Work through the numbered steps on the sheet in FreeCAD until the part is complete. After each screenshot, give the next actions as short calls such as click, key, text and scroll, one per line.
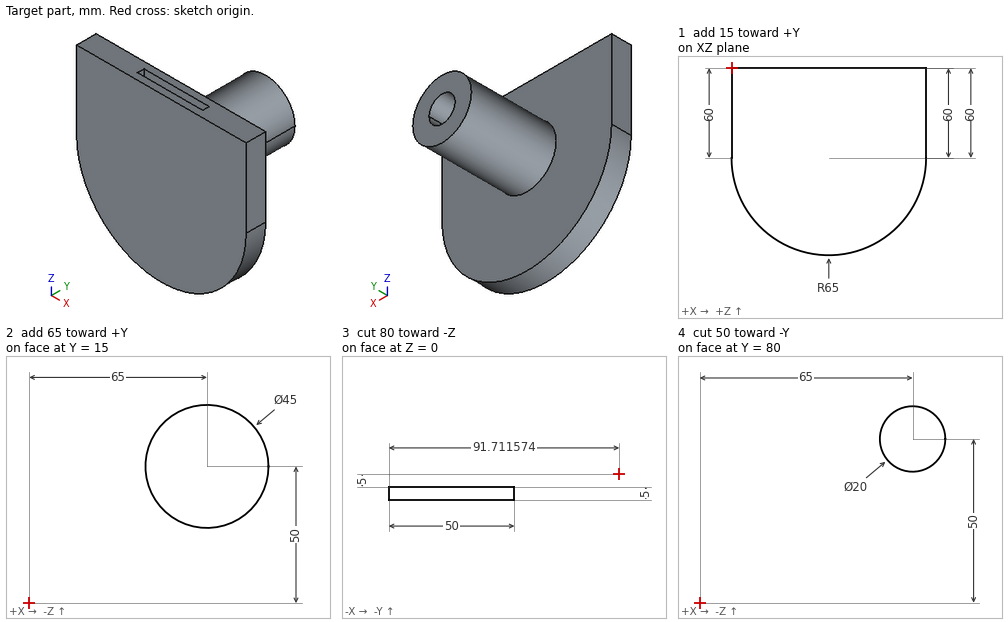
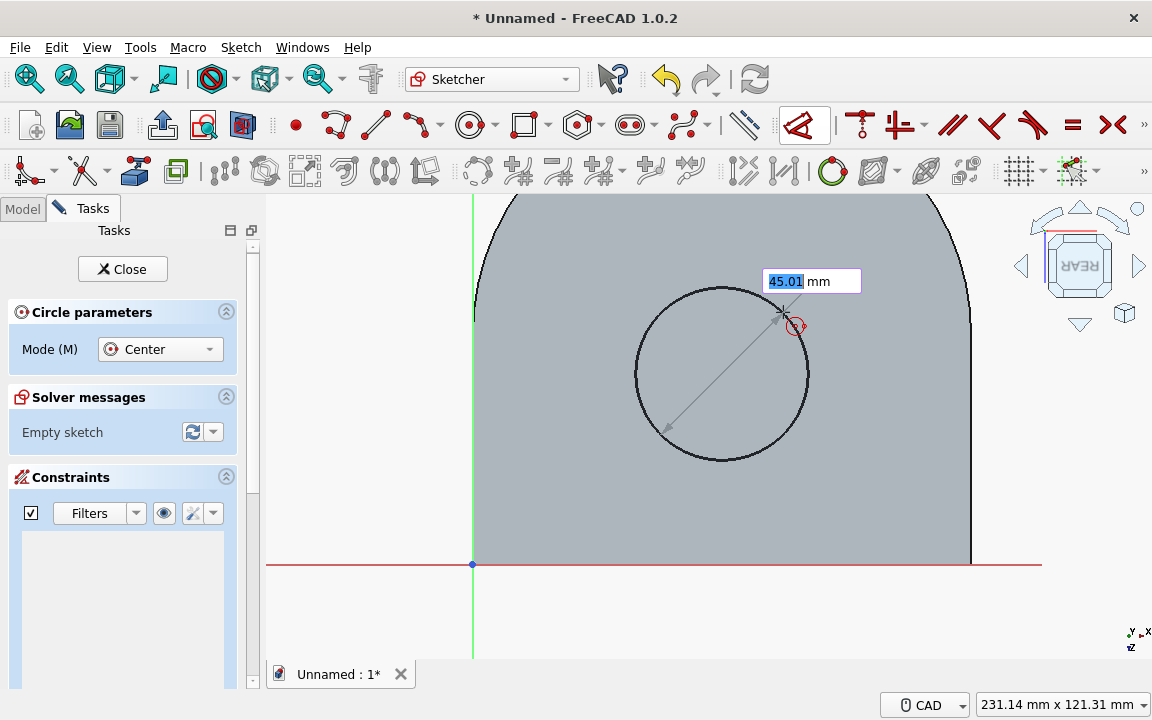
text(45)
key(Return)
key(Escape)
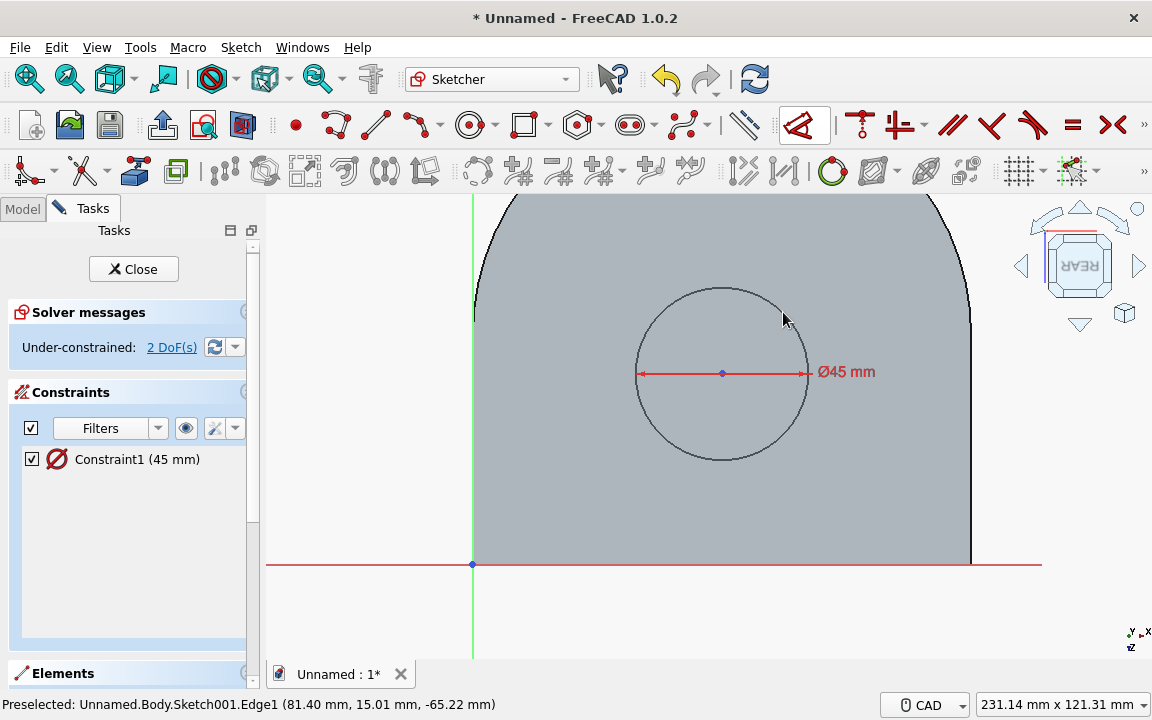
click(722, 374)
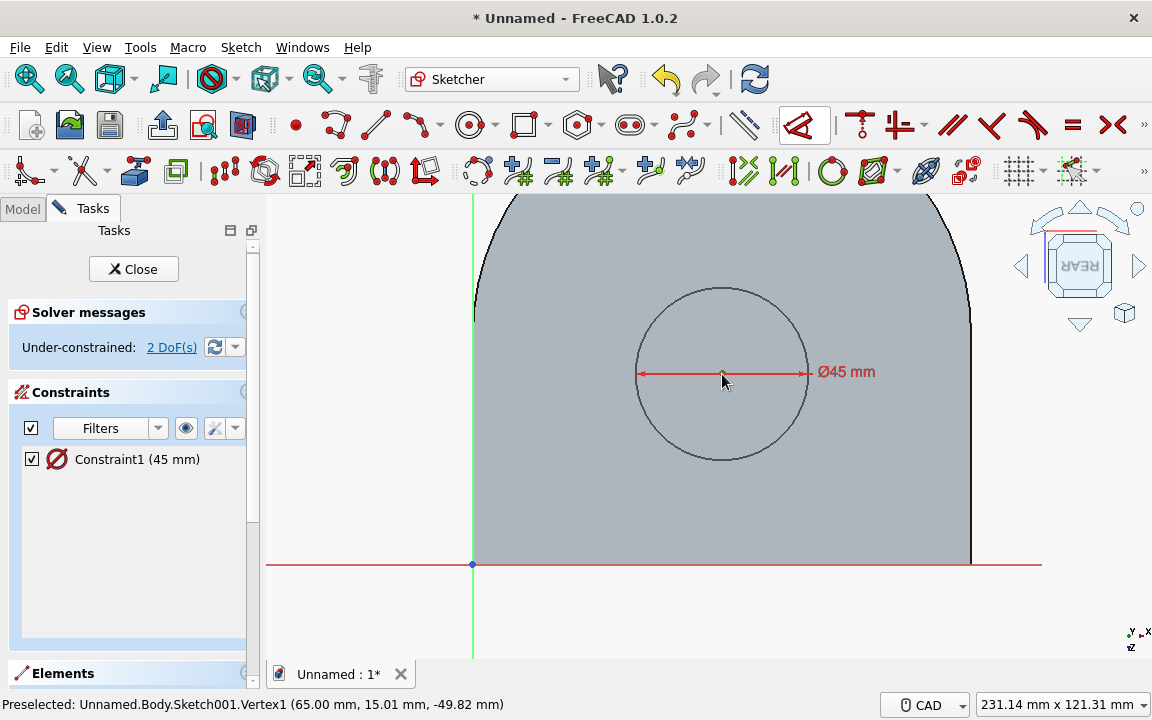
click(824, 126)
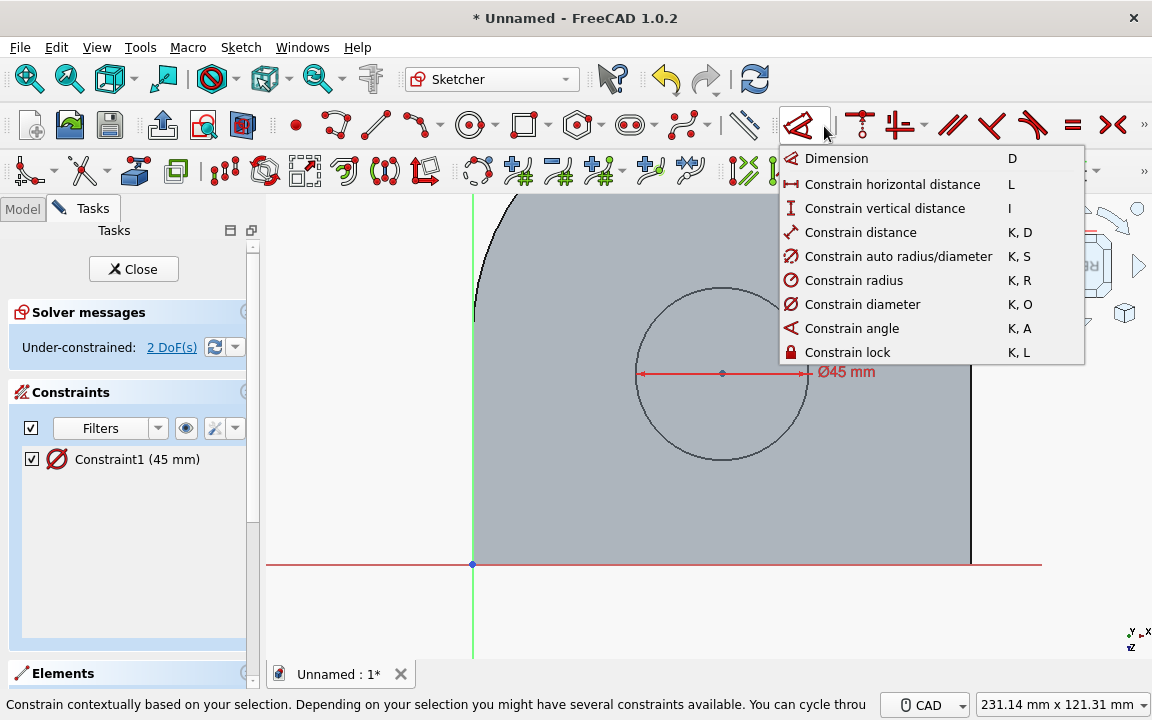
click(932, 184)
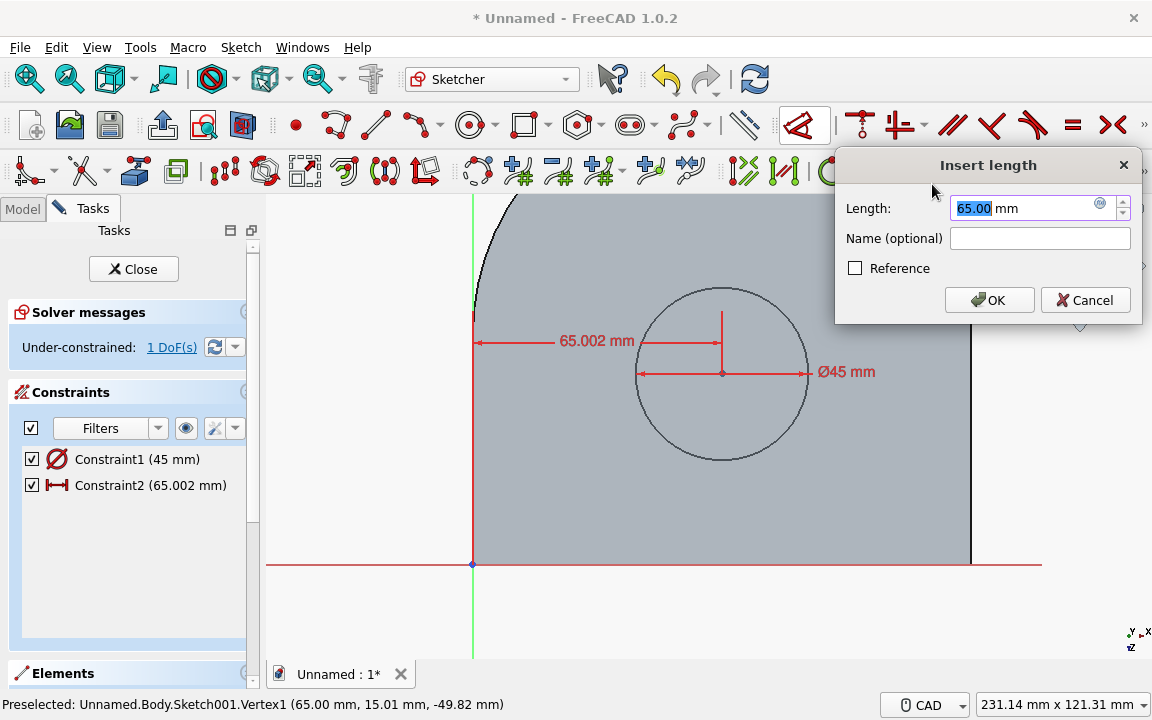
text(65)
key(Return)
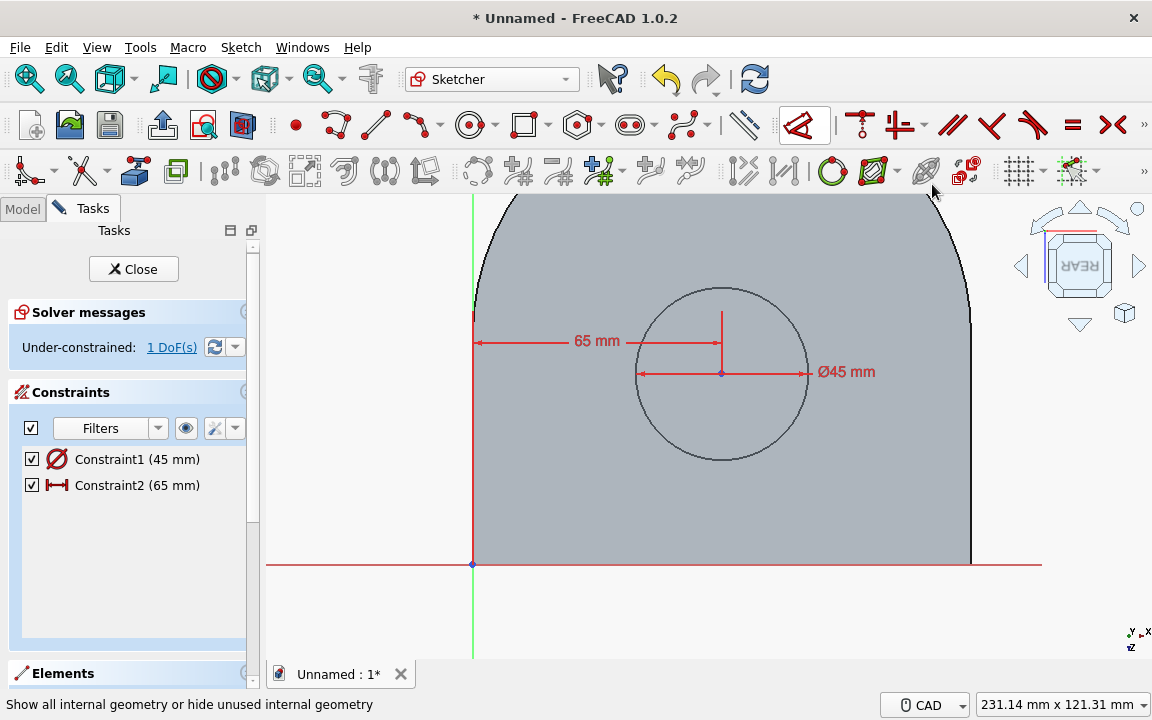
click(722, 374)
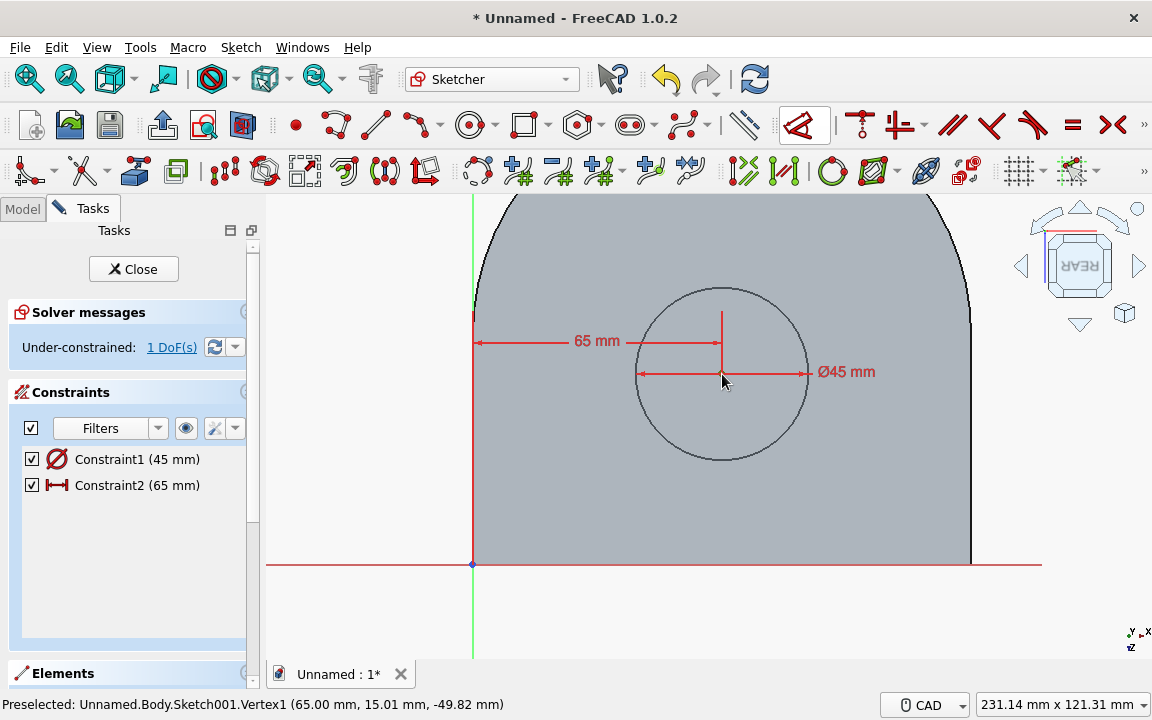
click(824, 126)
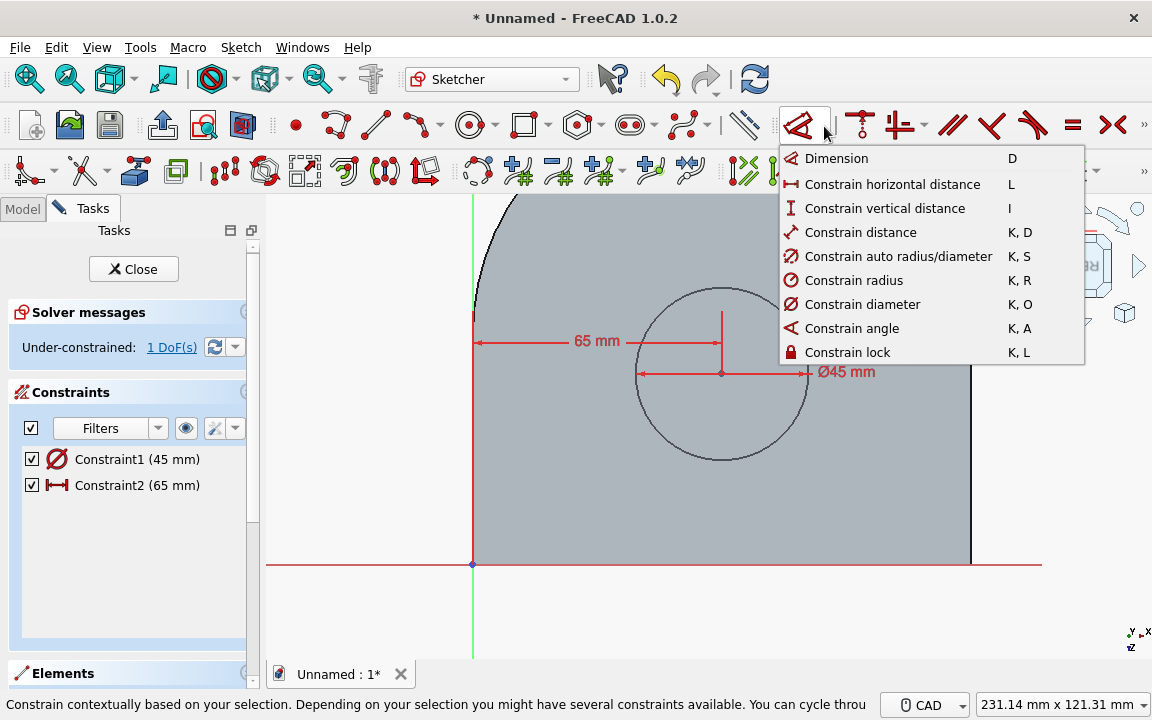
click(932, 208)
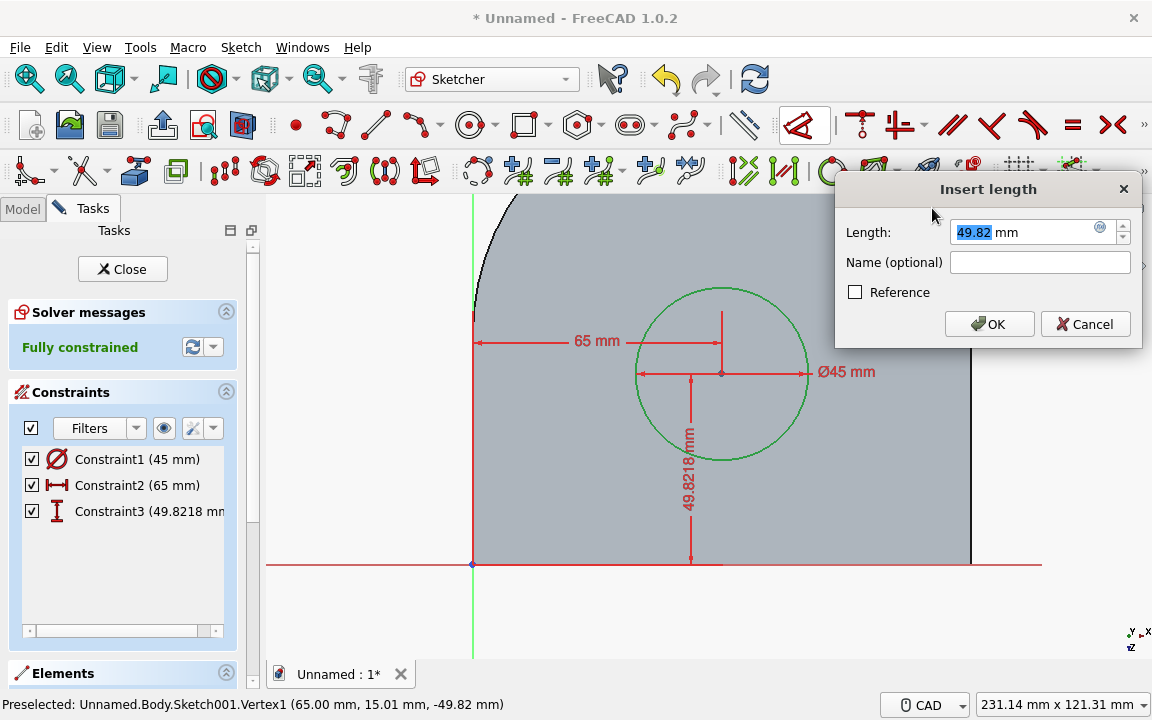
text(50)
key(Return)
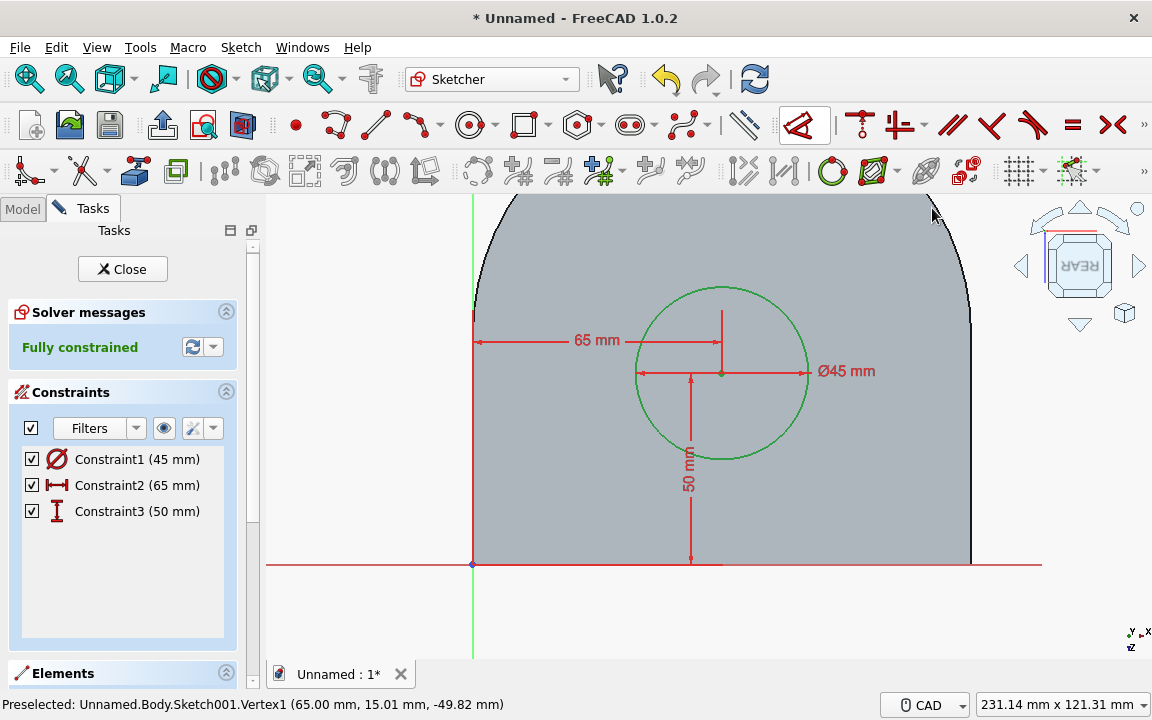
click(123, 269)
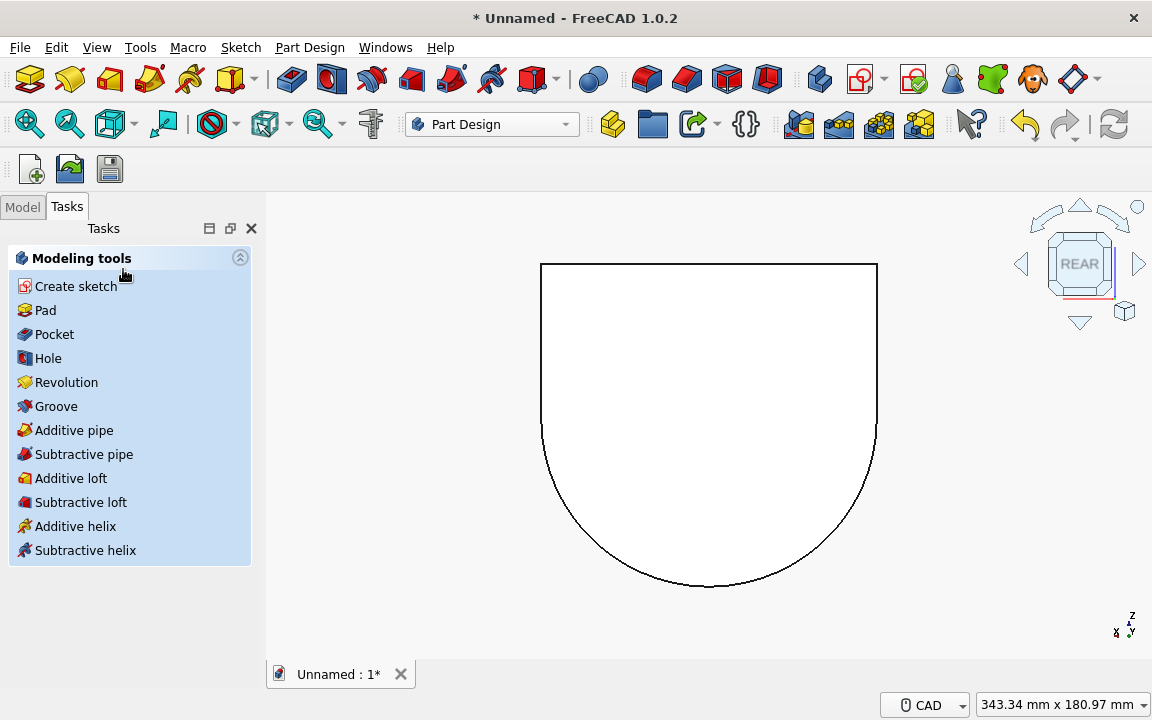
click(30, 80)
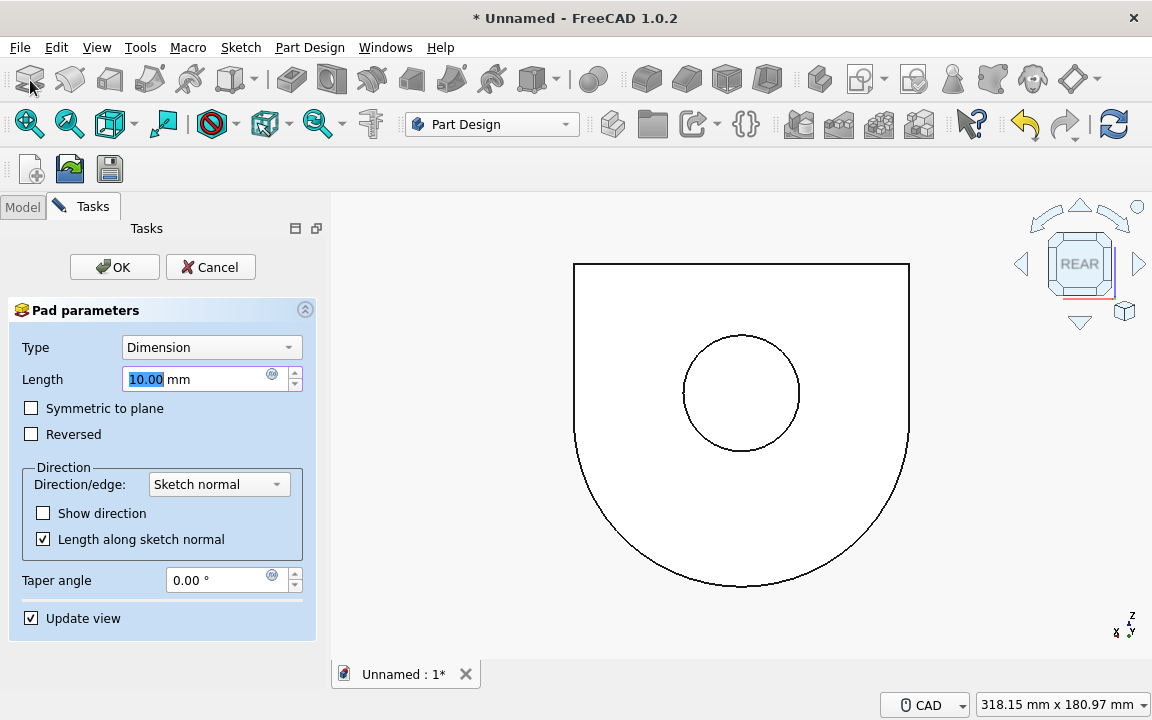
text(65)
key(Tab)